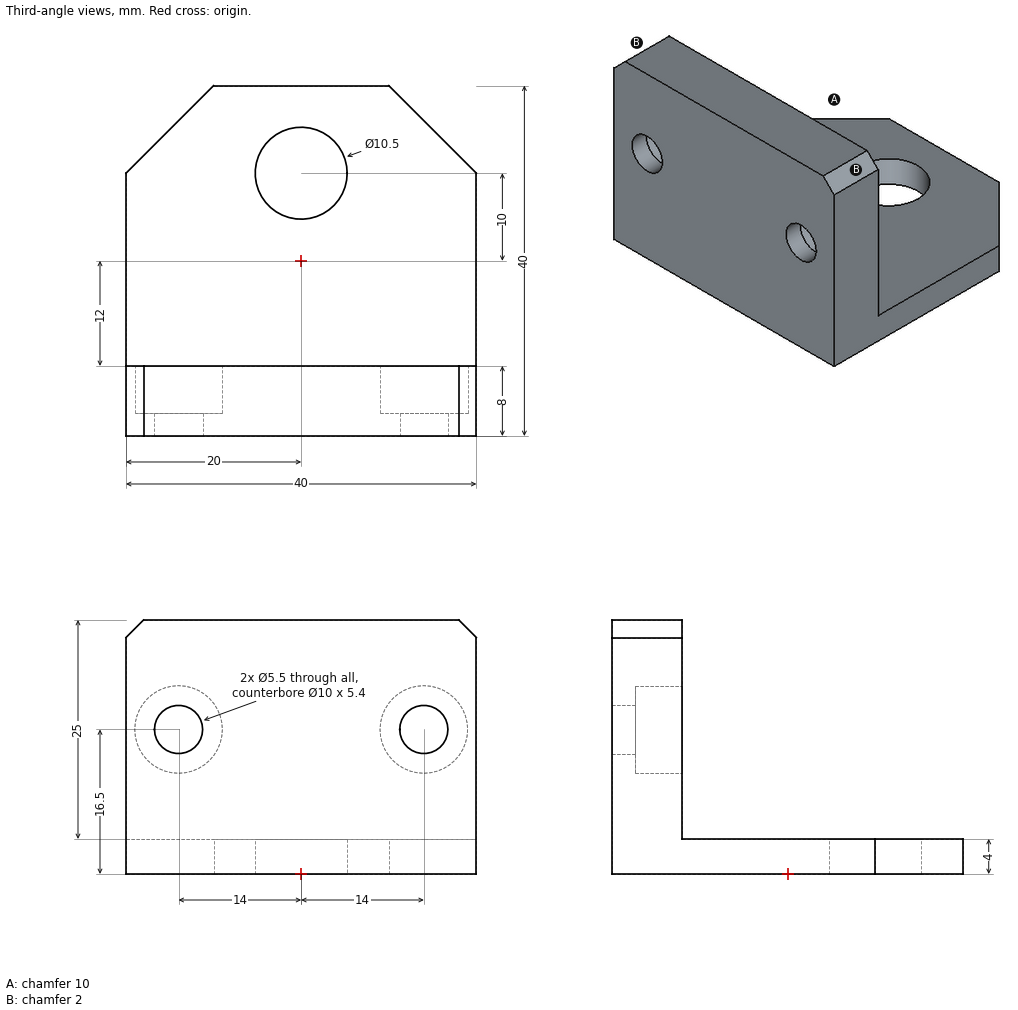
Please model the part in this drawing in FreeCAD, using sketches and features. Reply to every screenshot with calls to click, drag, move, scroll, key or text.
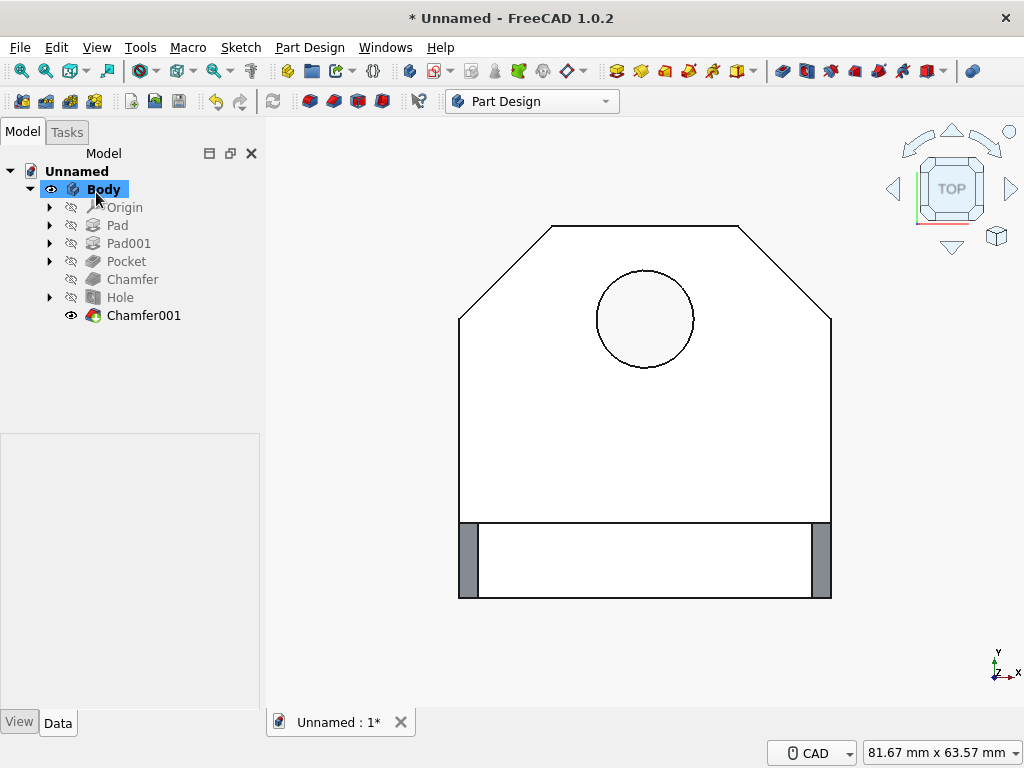
key(0)